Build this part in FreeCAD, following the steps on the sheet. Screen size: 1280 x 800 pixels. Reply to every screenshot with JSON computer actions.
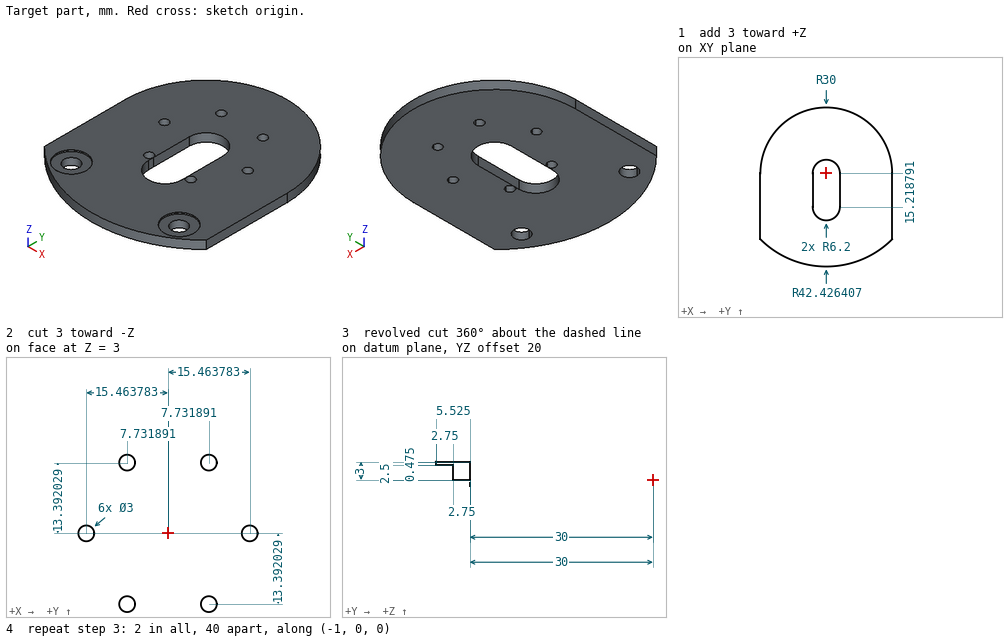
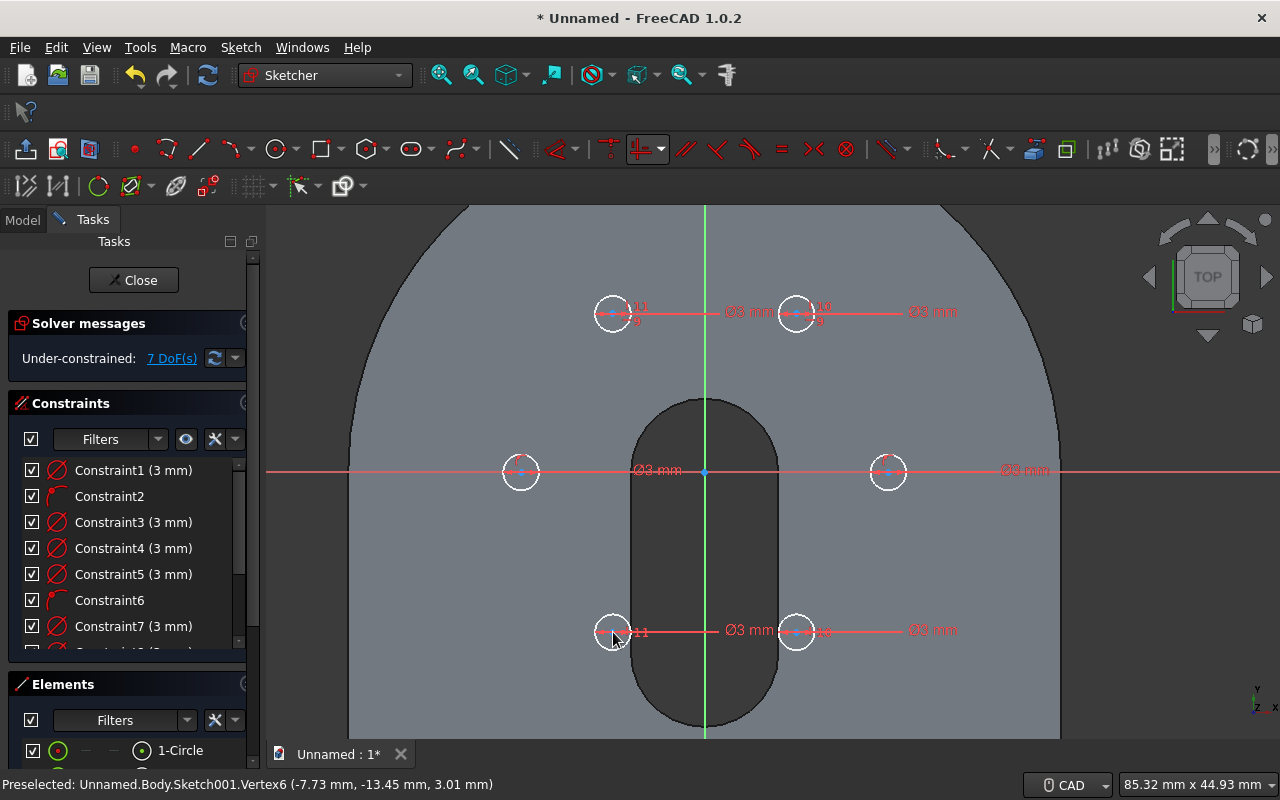
{"action": "left_click", "coordinate": [797, 632]}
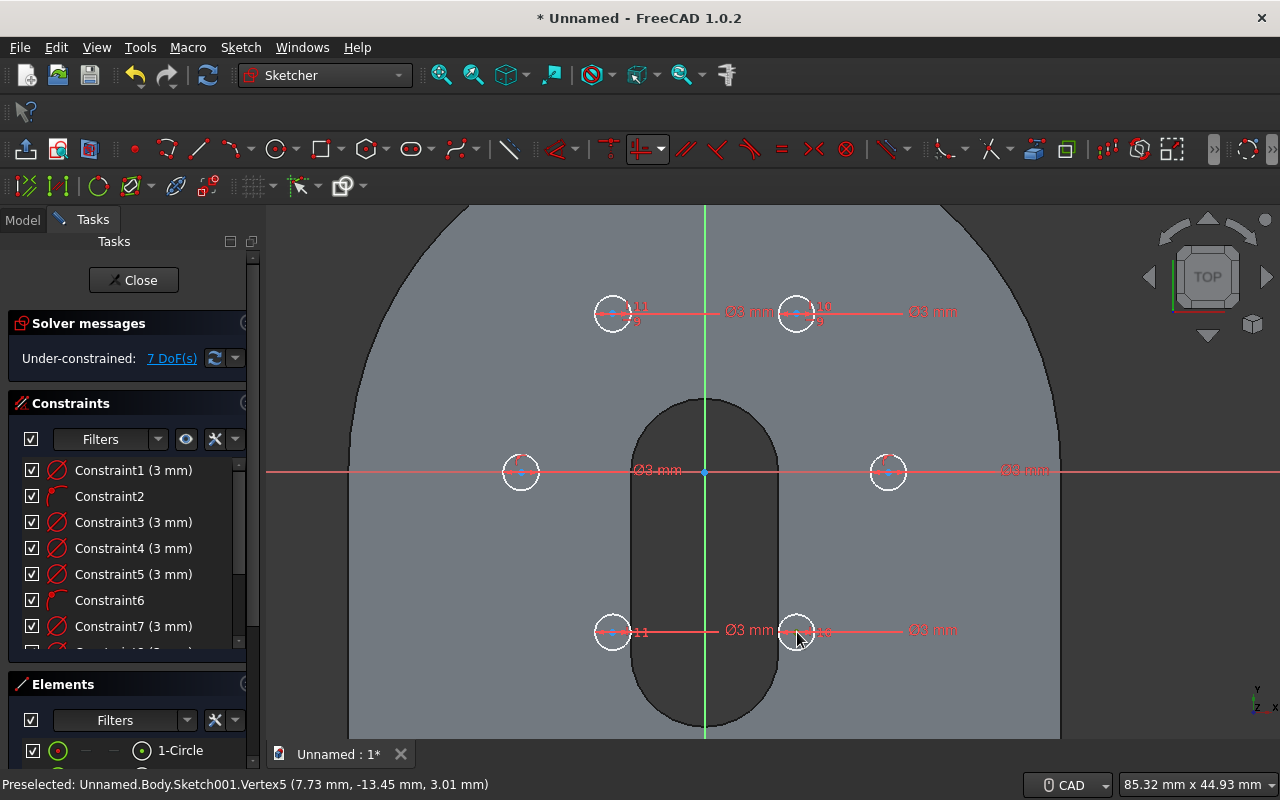
{"action": "left_click", "coordinate": [613, 632]}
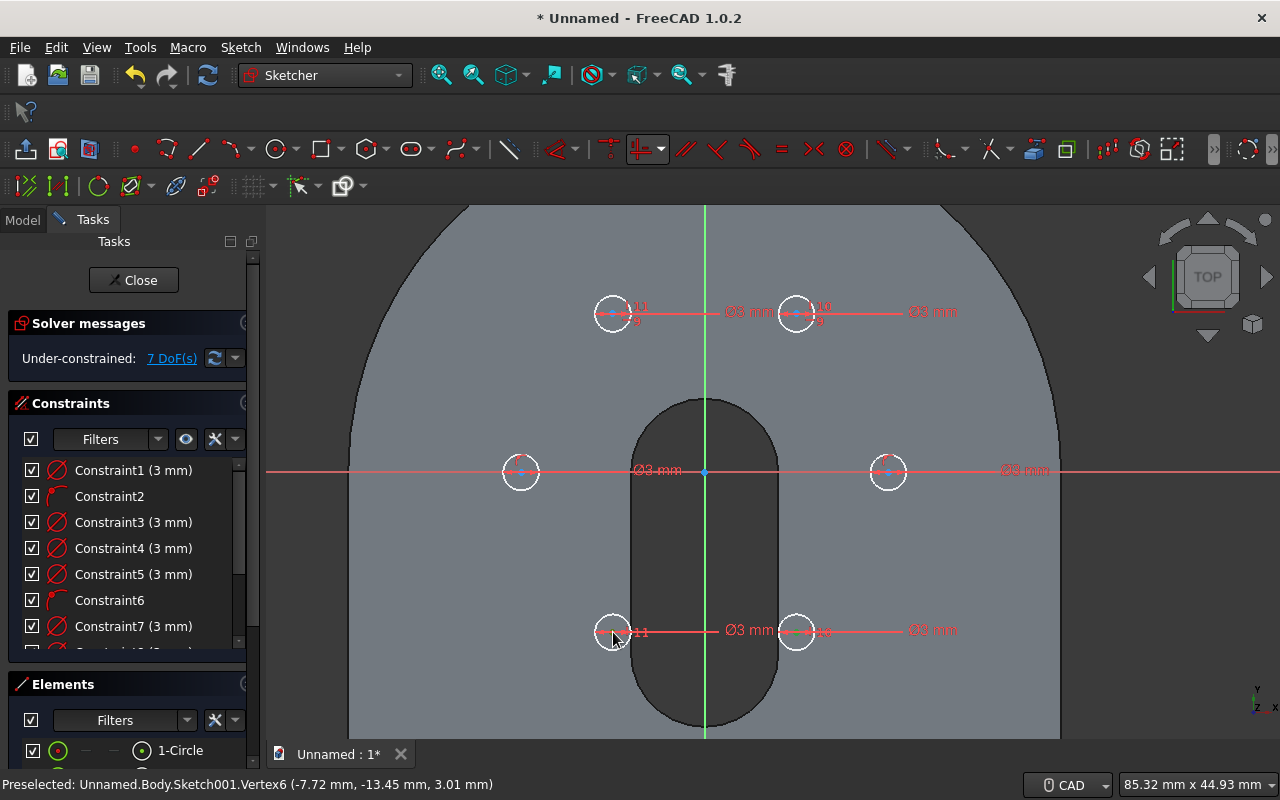
{"action": "left_click", "coordinate": [664, 150]}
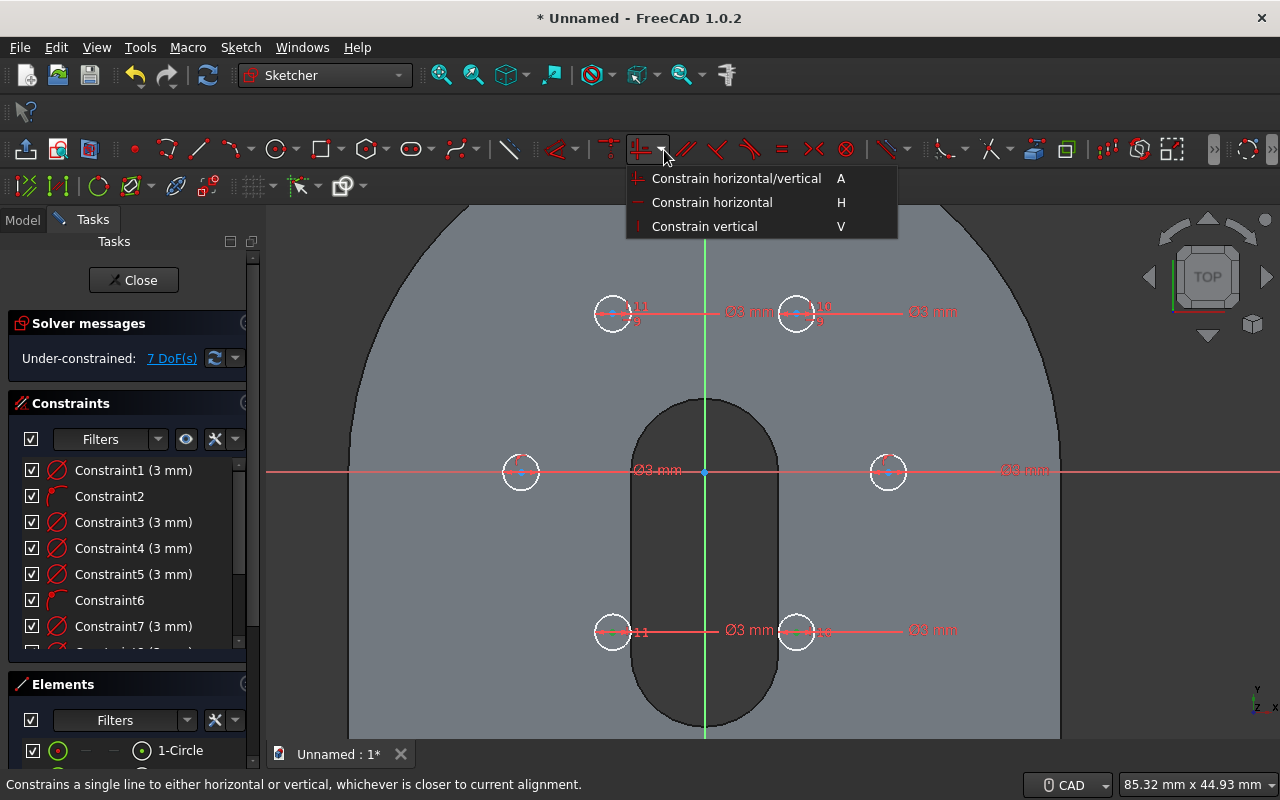
{"action": "left_click", "coordinate": [762, 202]}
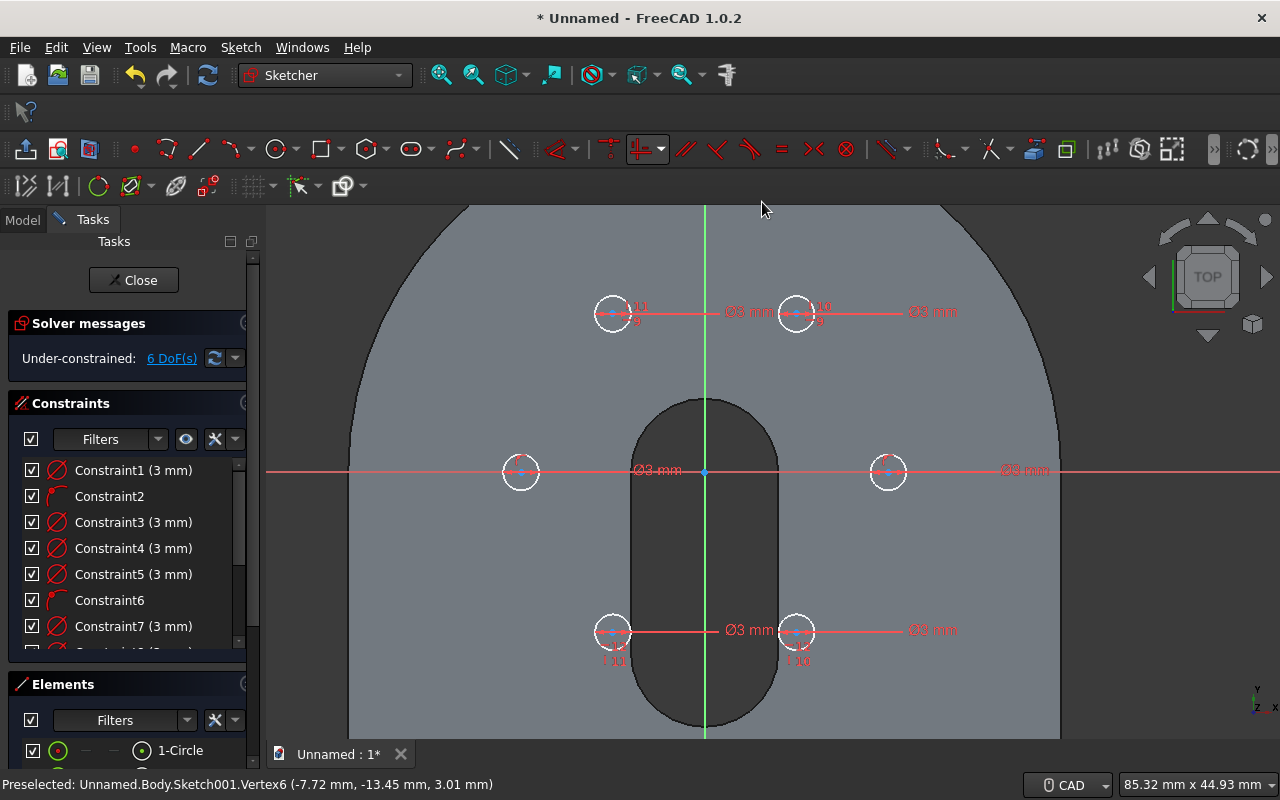
{"action": "left_click", "coordinate": [556, 150]}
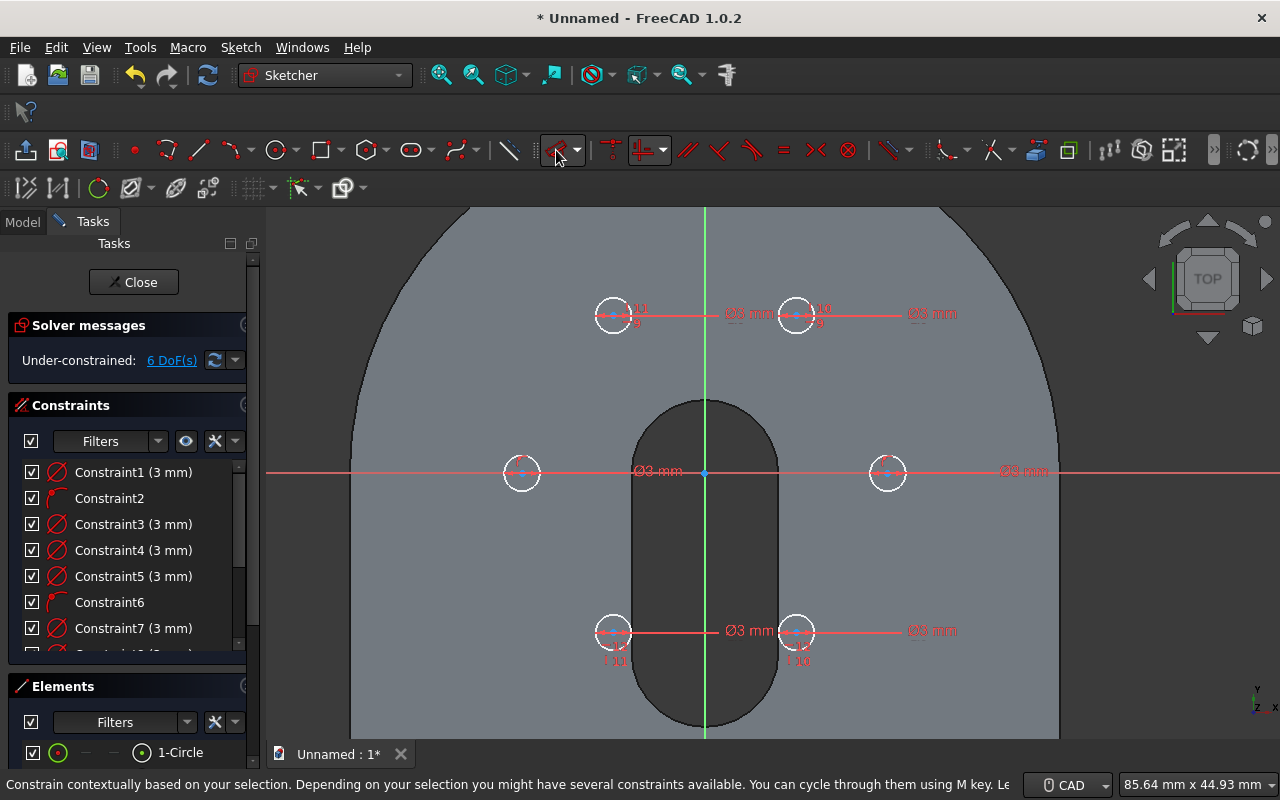
{"action": "left_click", "coordinate": [614, 316]}
{"action": "left_click", "coordinate": [659, 282]}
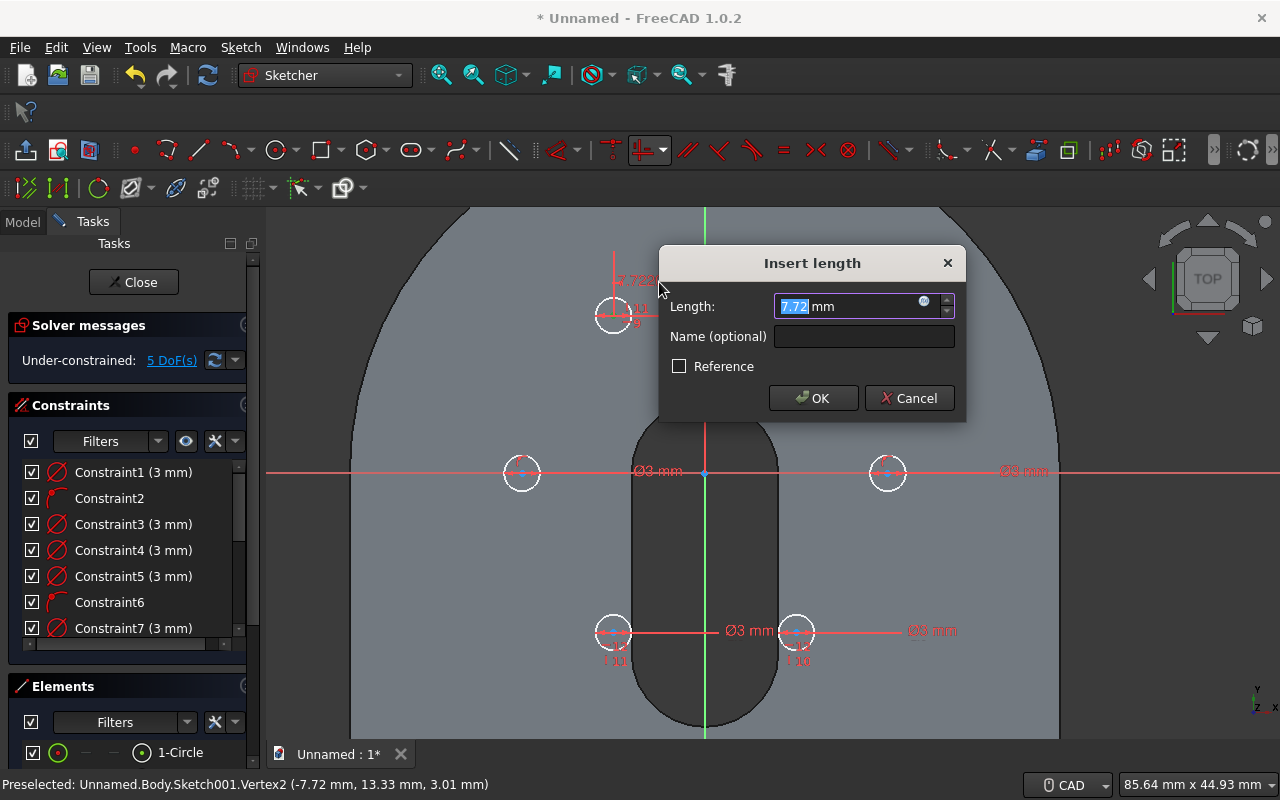
{"action": "type", "text": "7.731891"}
{"action": "key", "text": "Return"}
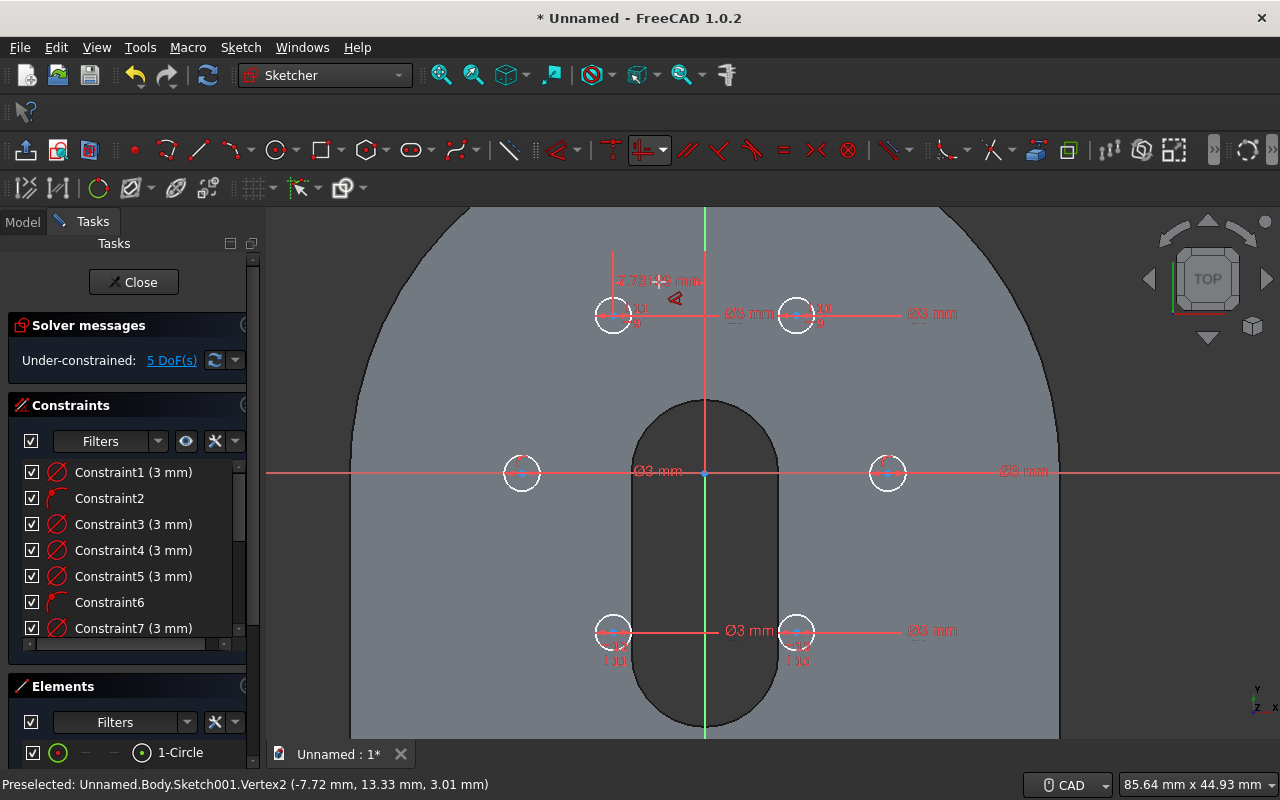
{"action": "left_click", "coordinate": [796, 316]}
{"action": "left_click", "coordinate": [751, 282]}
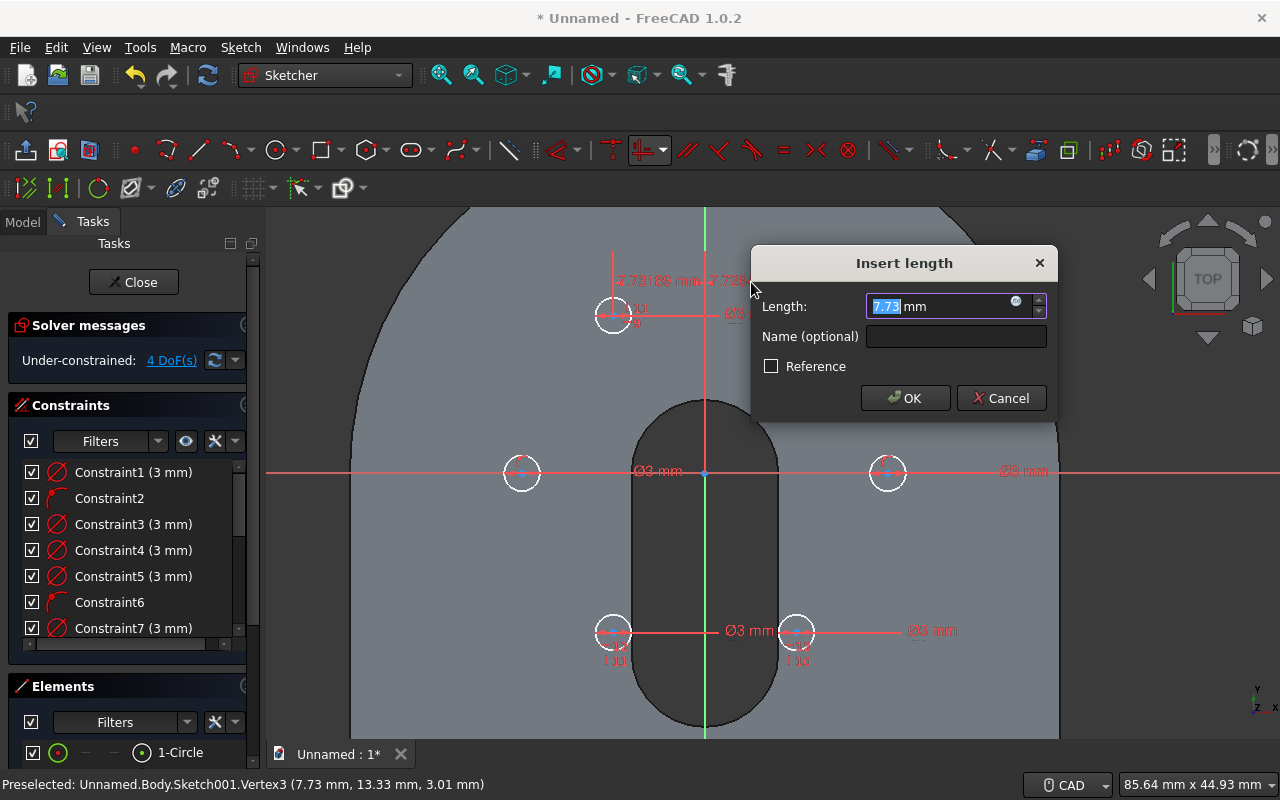
{"action": "type", "text": "7.731891"}
{"action": "key", "text": "Return"}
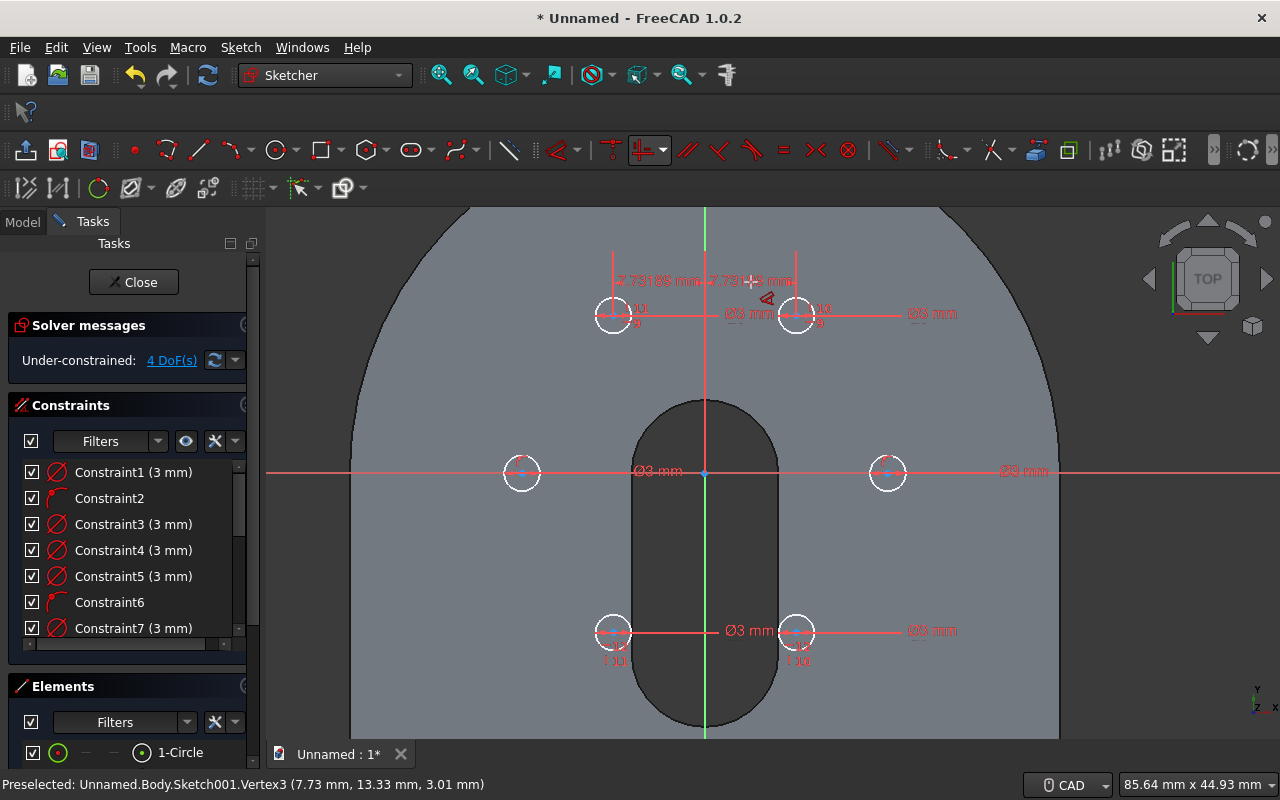
{"action": "left_click", "coordinate": [522, 473]}
{"action": "left_click", "coordinate": [613, 507]}